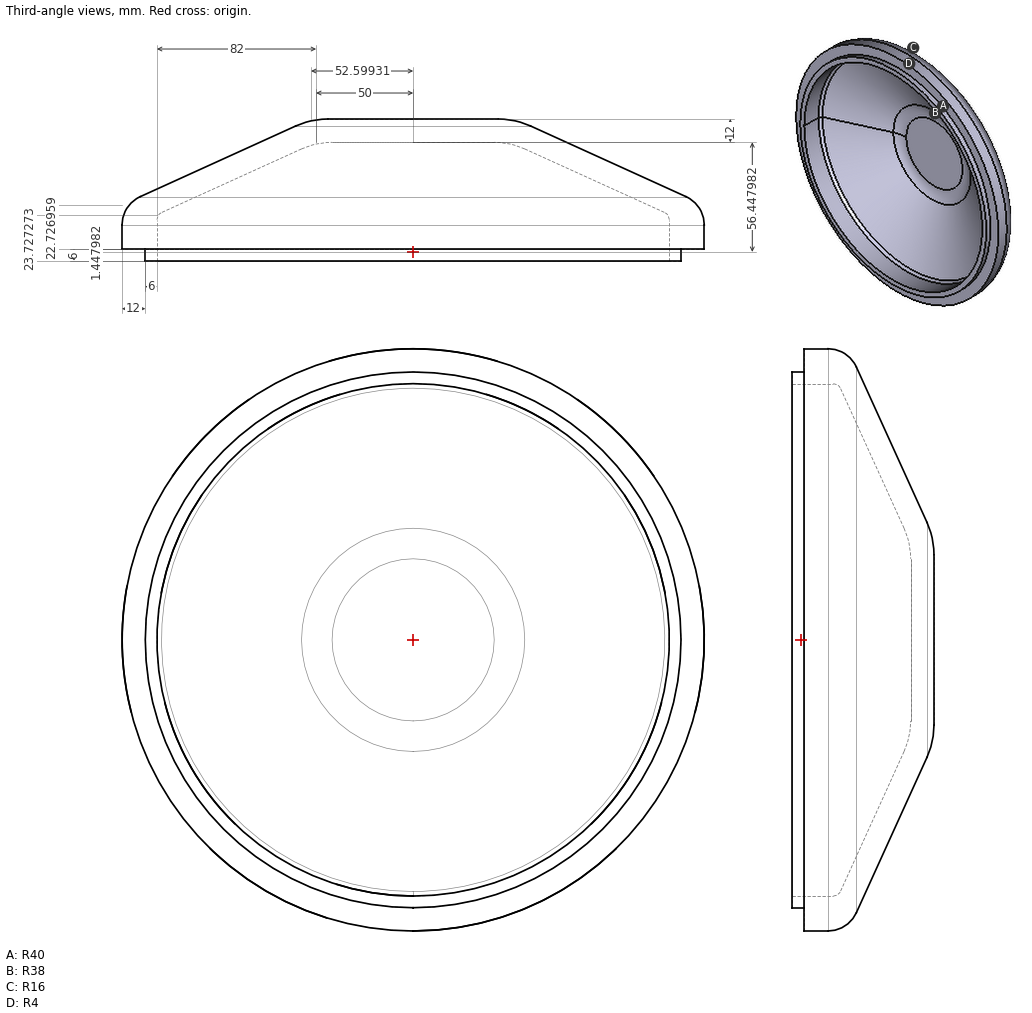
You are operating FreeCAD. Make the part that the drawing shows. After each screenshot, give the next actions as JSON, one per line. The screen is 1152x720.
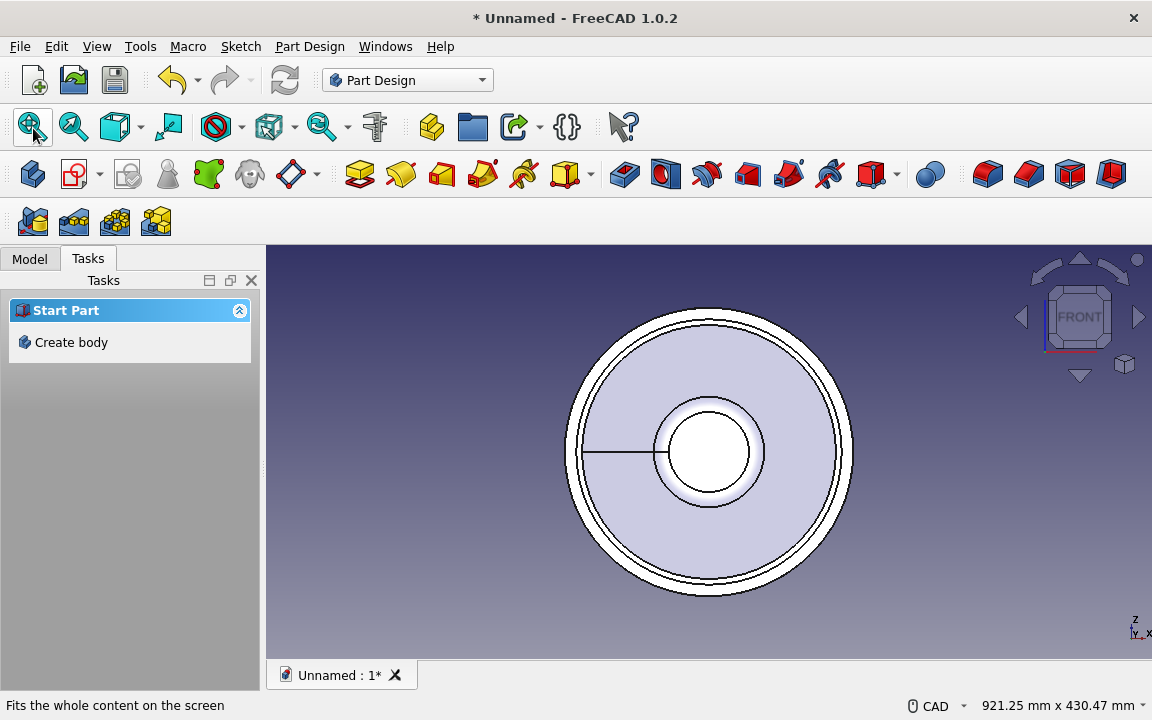
{"action": "key", "text": "3"}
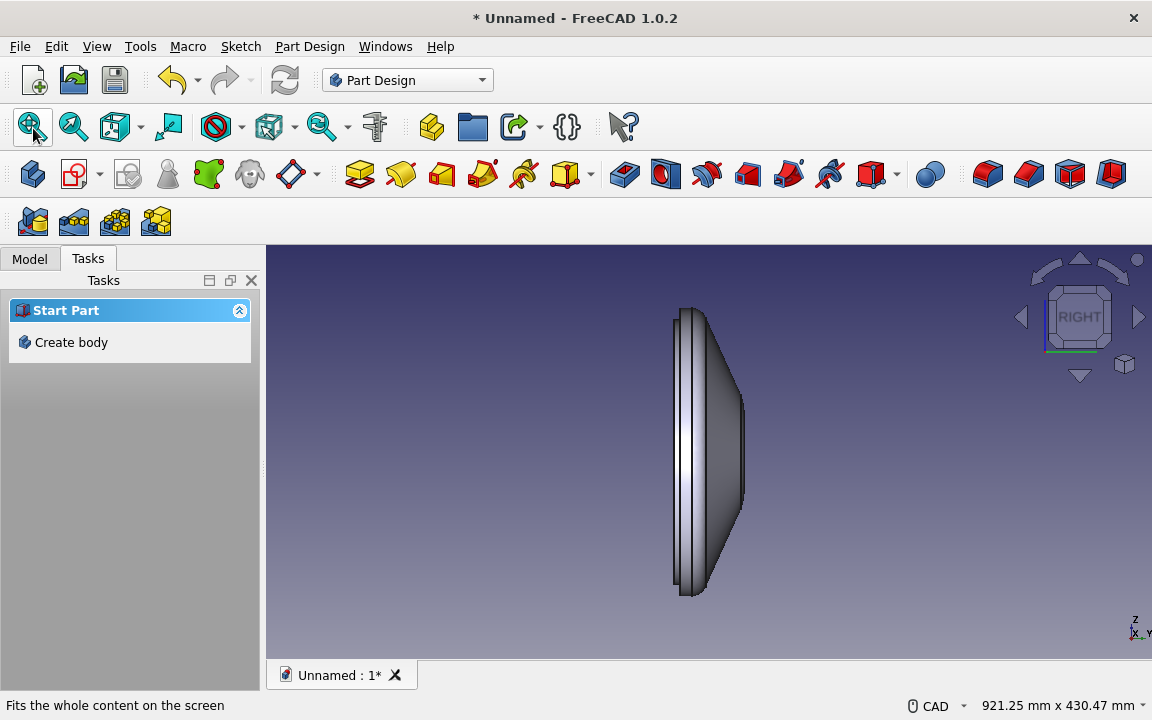
{"action": "key", "text": "5"}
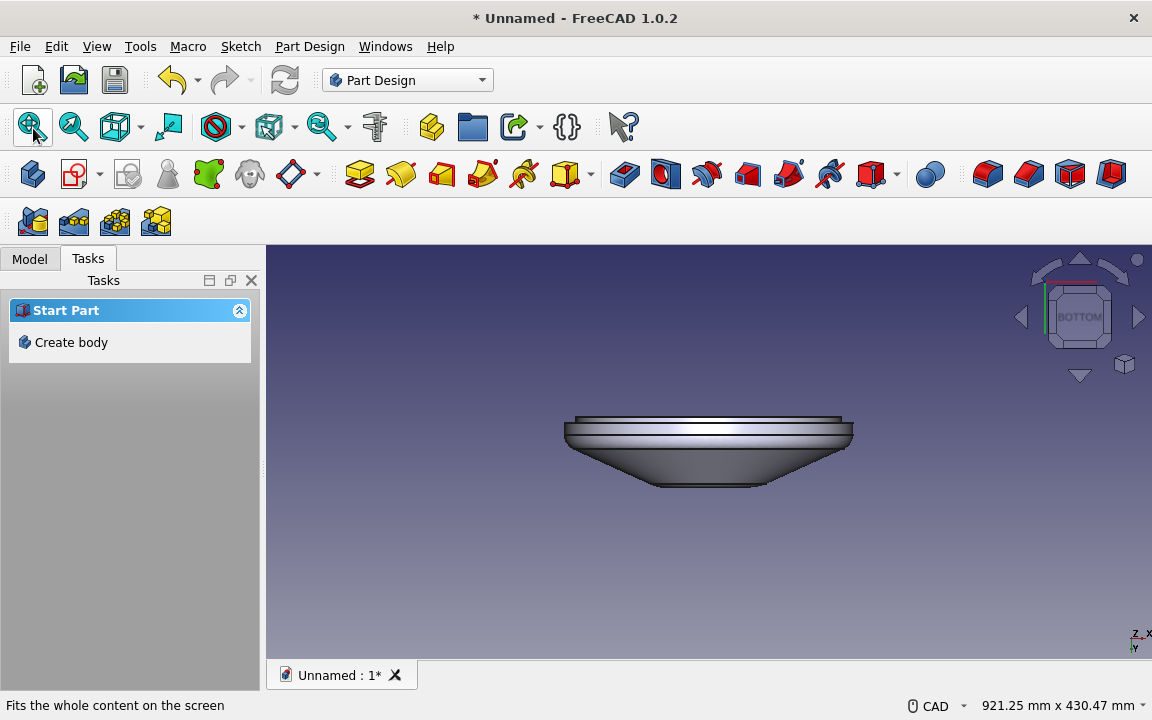
{"action": "key", "text": "v f"}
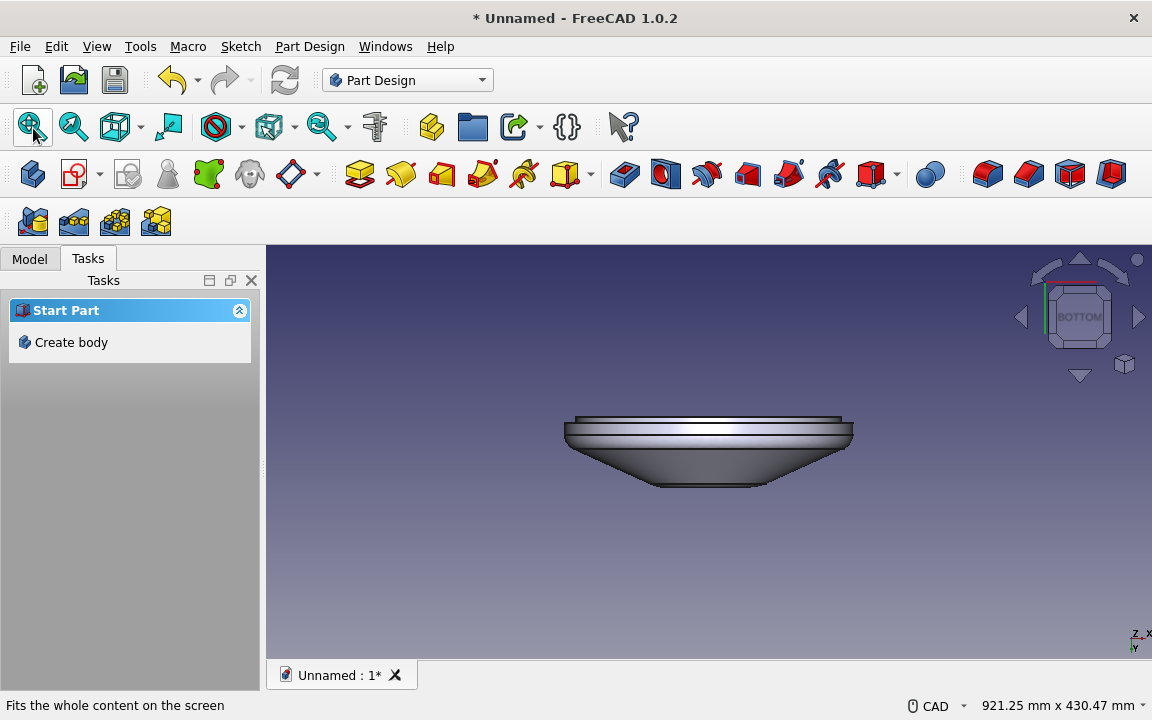
{"action": "key", "text": "4"}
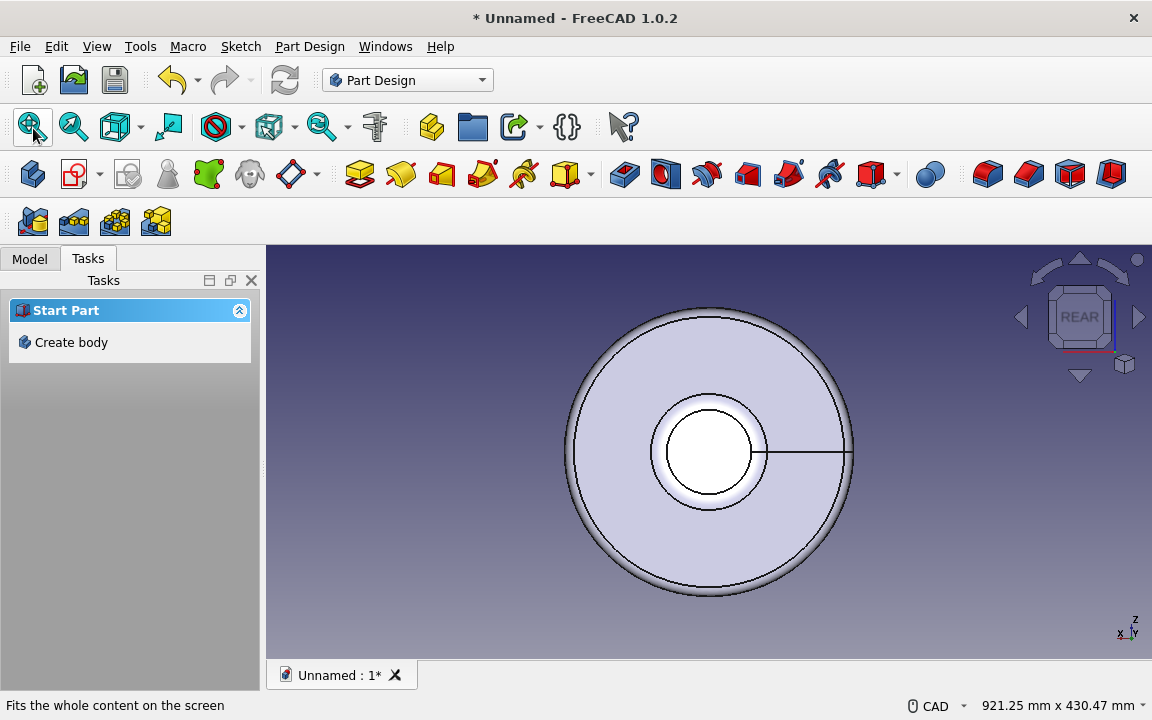
{"action": "key", "text": "6"}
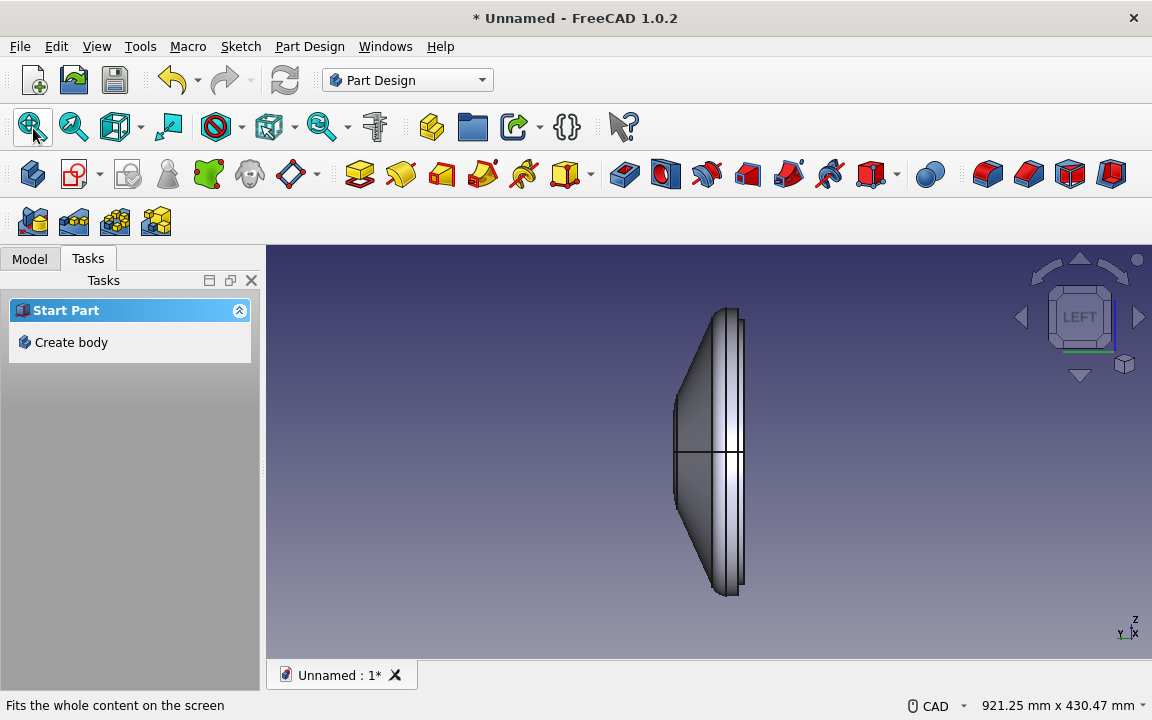
{"action": "key", "text": "v 3"}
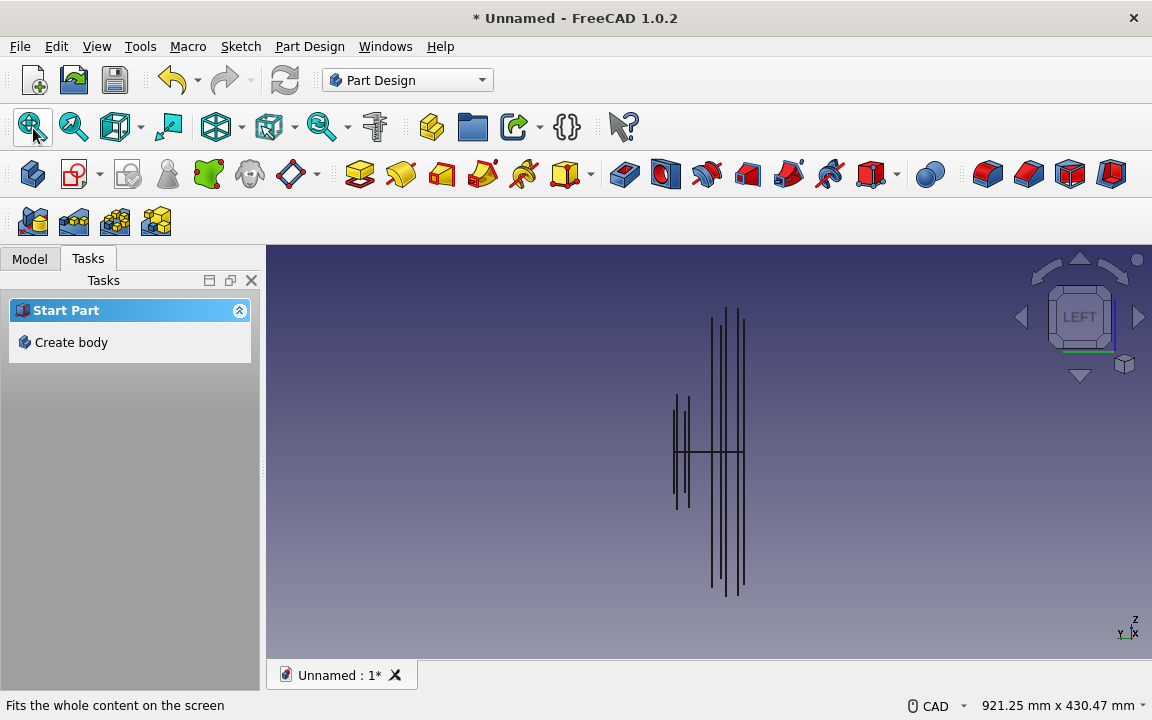
{"action": "key", "text": "0"}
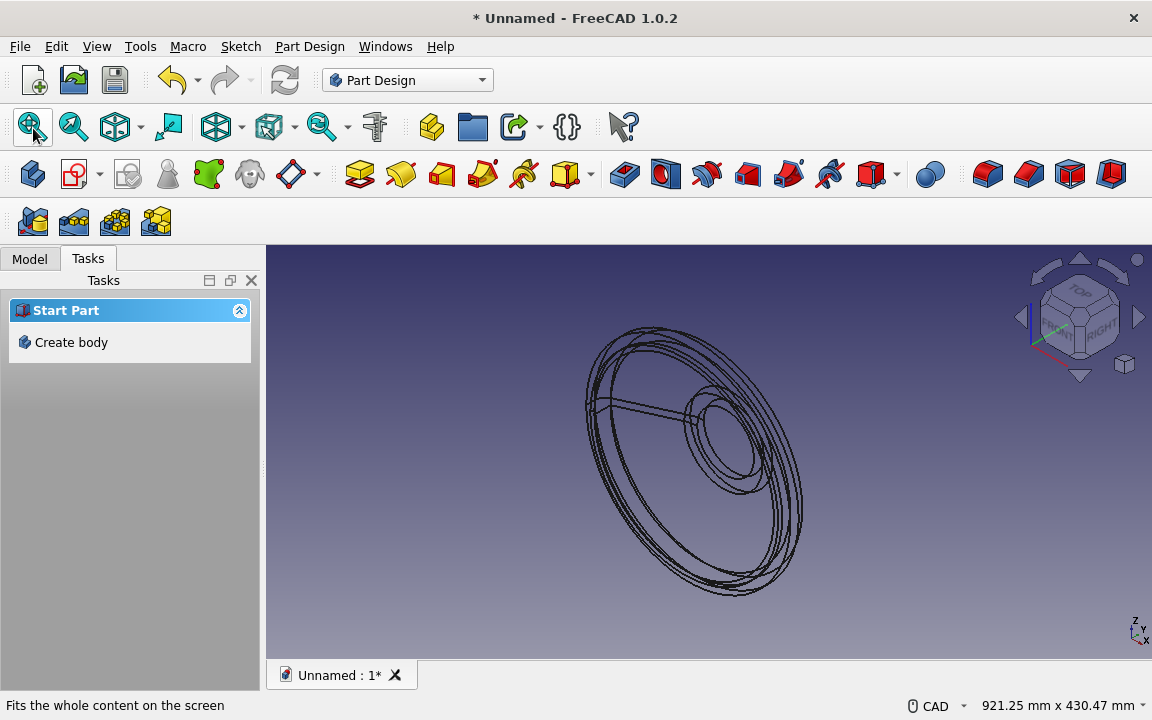
{"action": "left_click", "coordinate": [728, 571]}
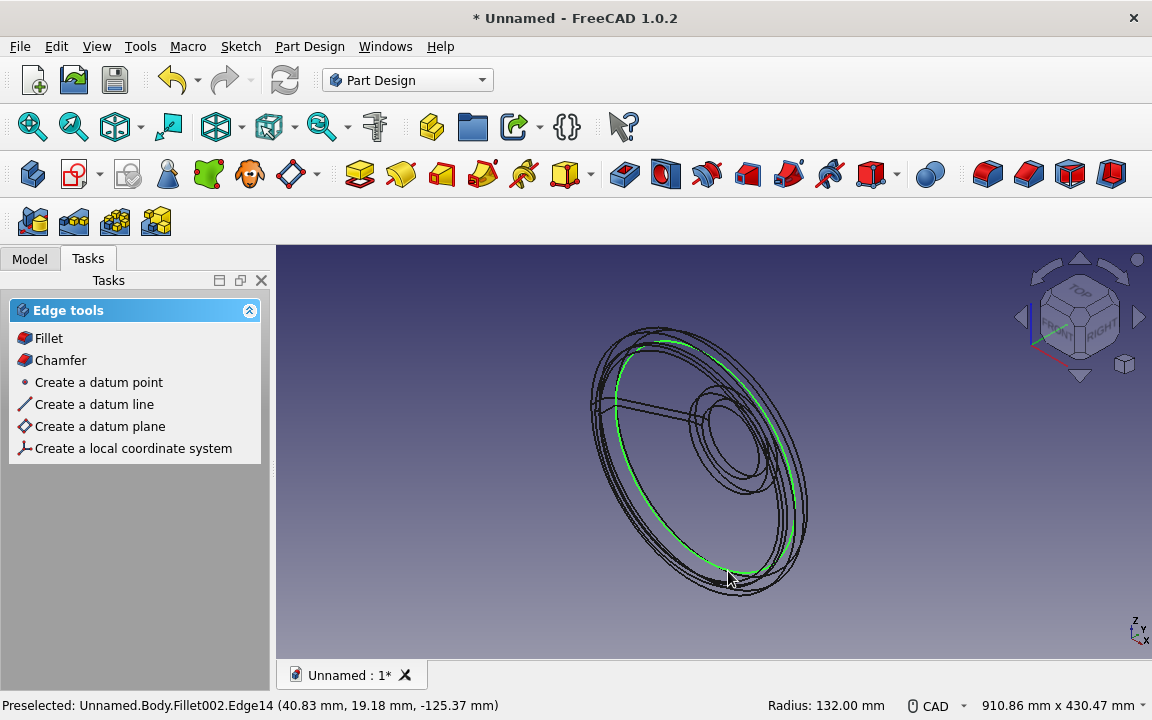
{"action": "key", "text": "v 1"}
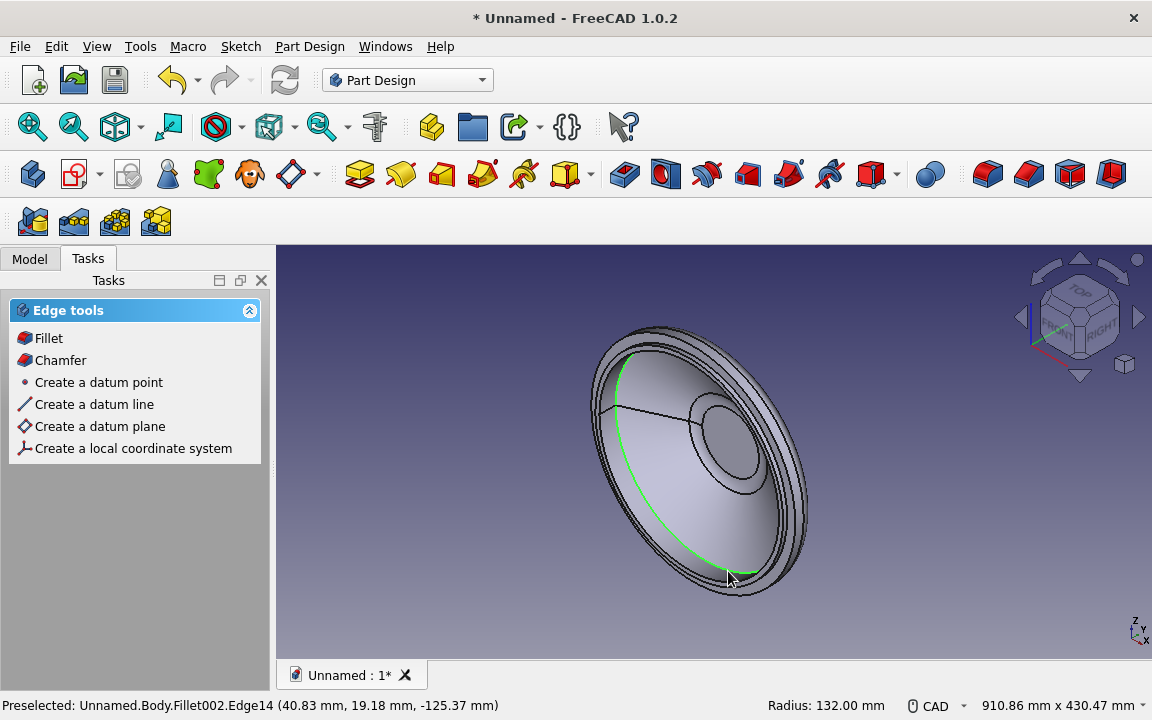
{"action": "left_click", "coordinate": [988, 174]}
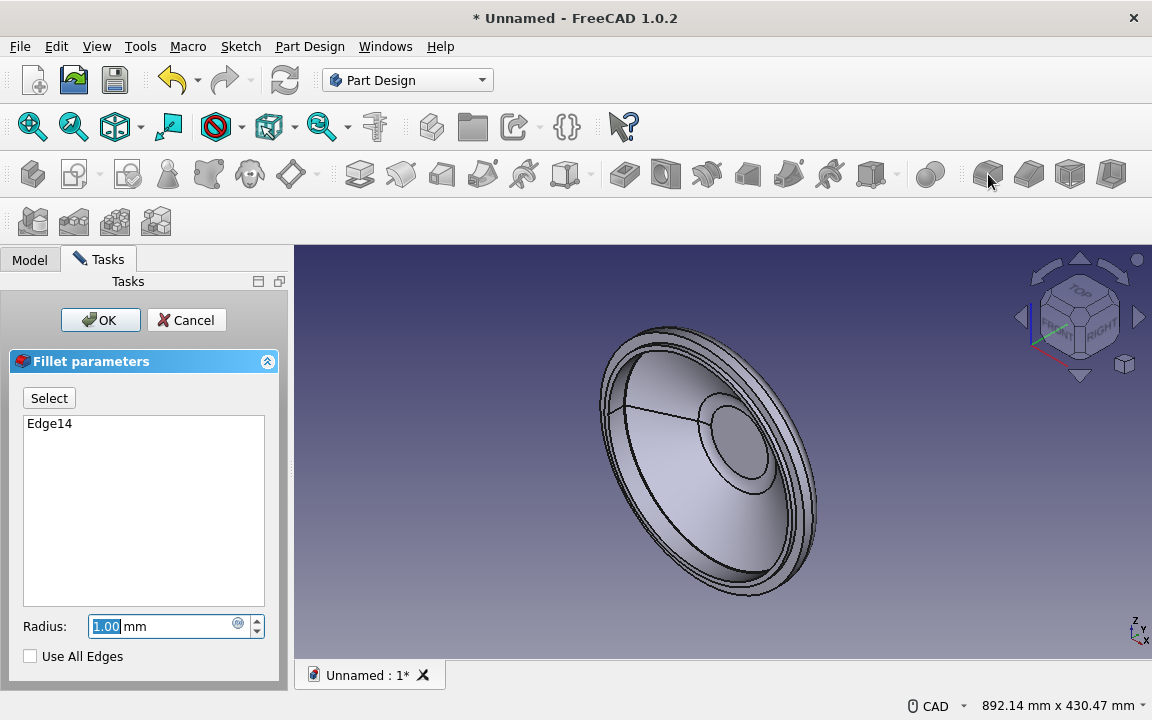
{"action": "type", "text": "4"}
{"action": "key", "text": "Tab"}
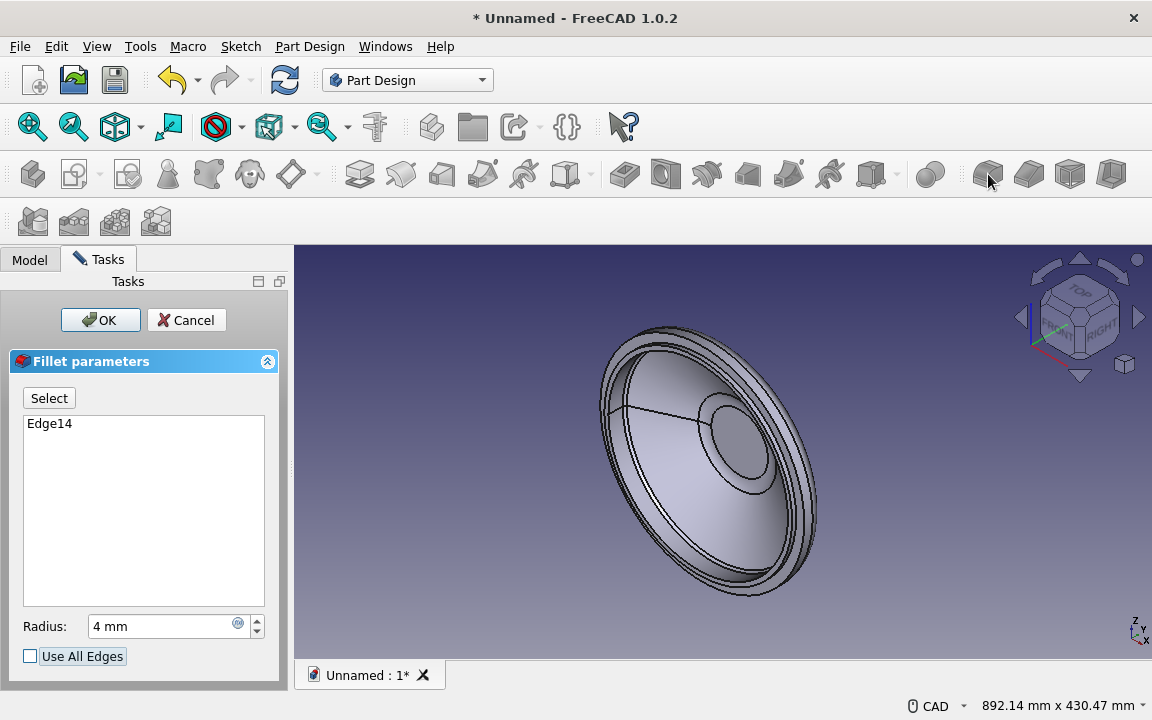
{"action": "left_click", "coordinate": [101, 320]}